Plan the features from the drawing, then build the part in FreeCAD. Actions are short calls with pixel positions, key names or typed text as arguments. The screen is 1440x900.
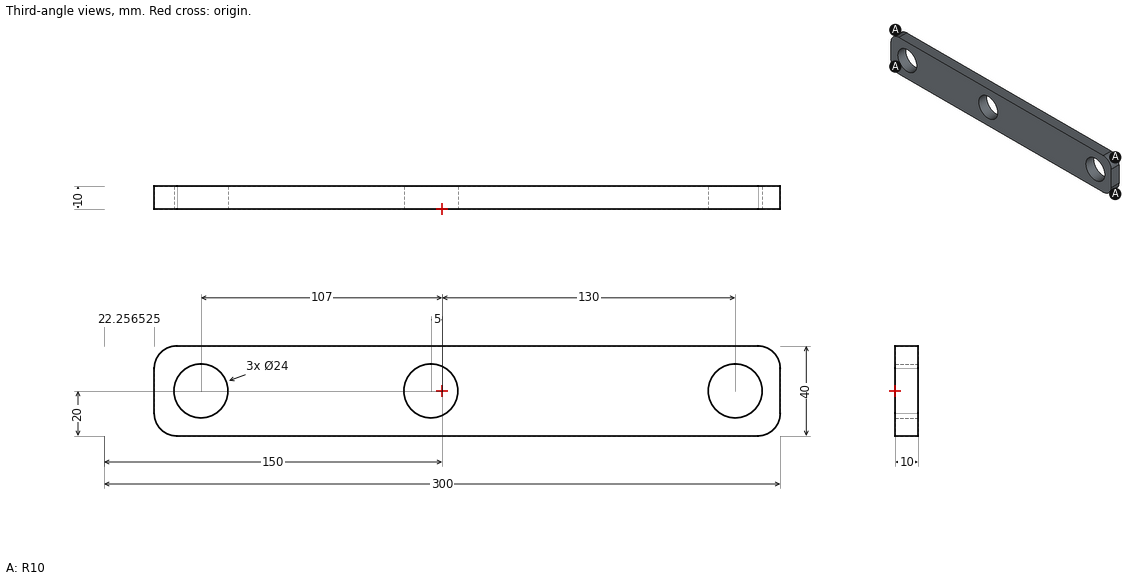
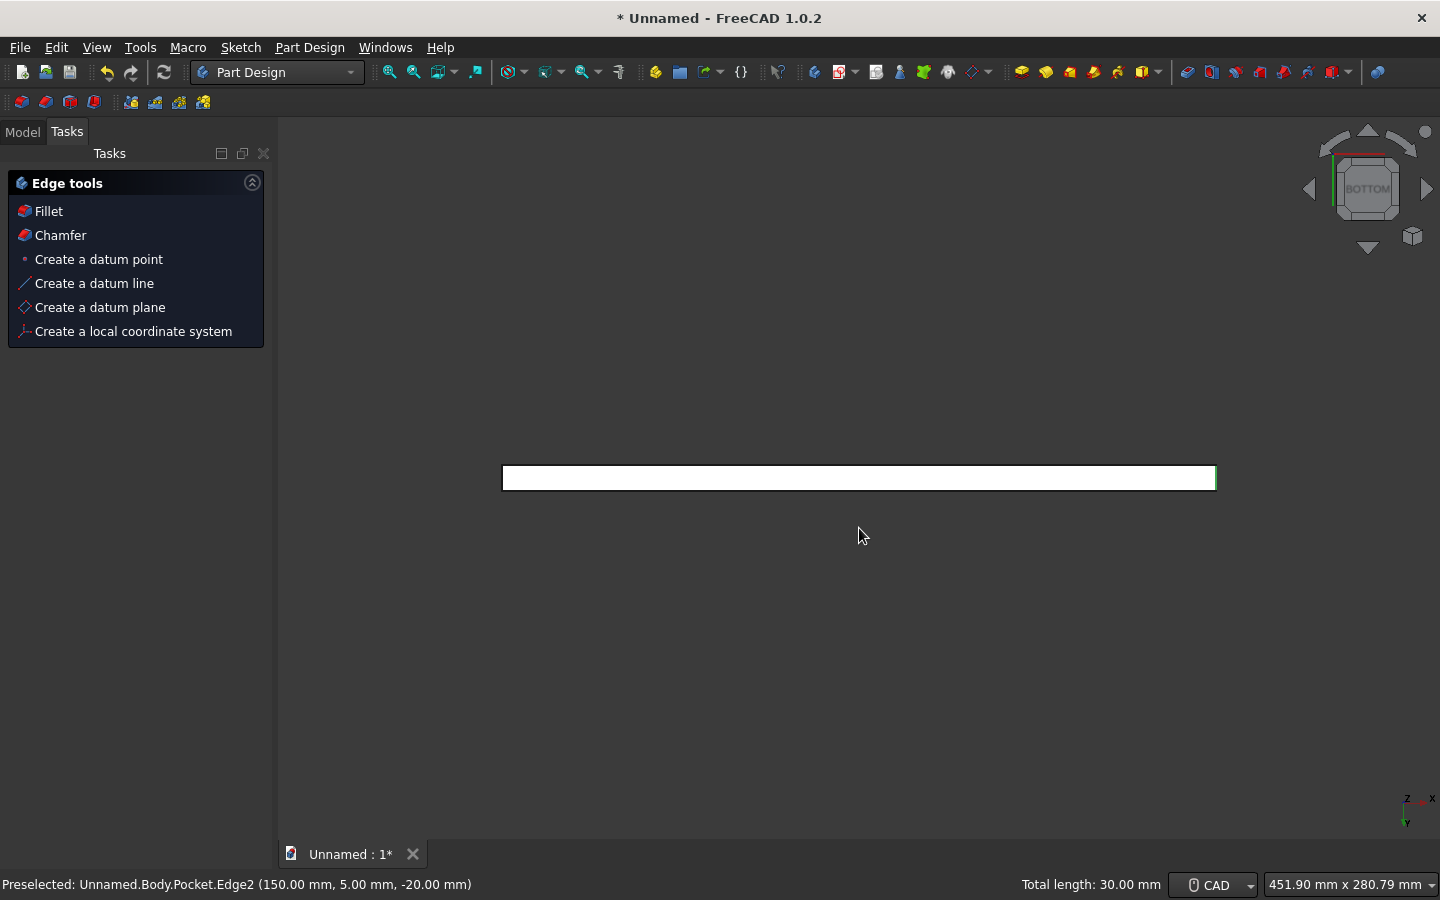
click(502, 477, ctrl)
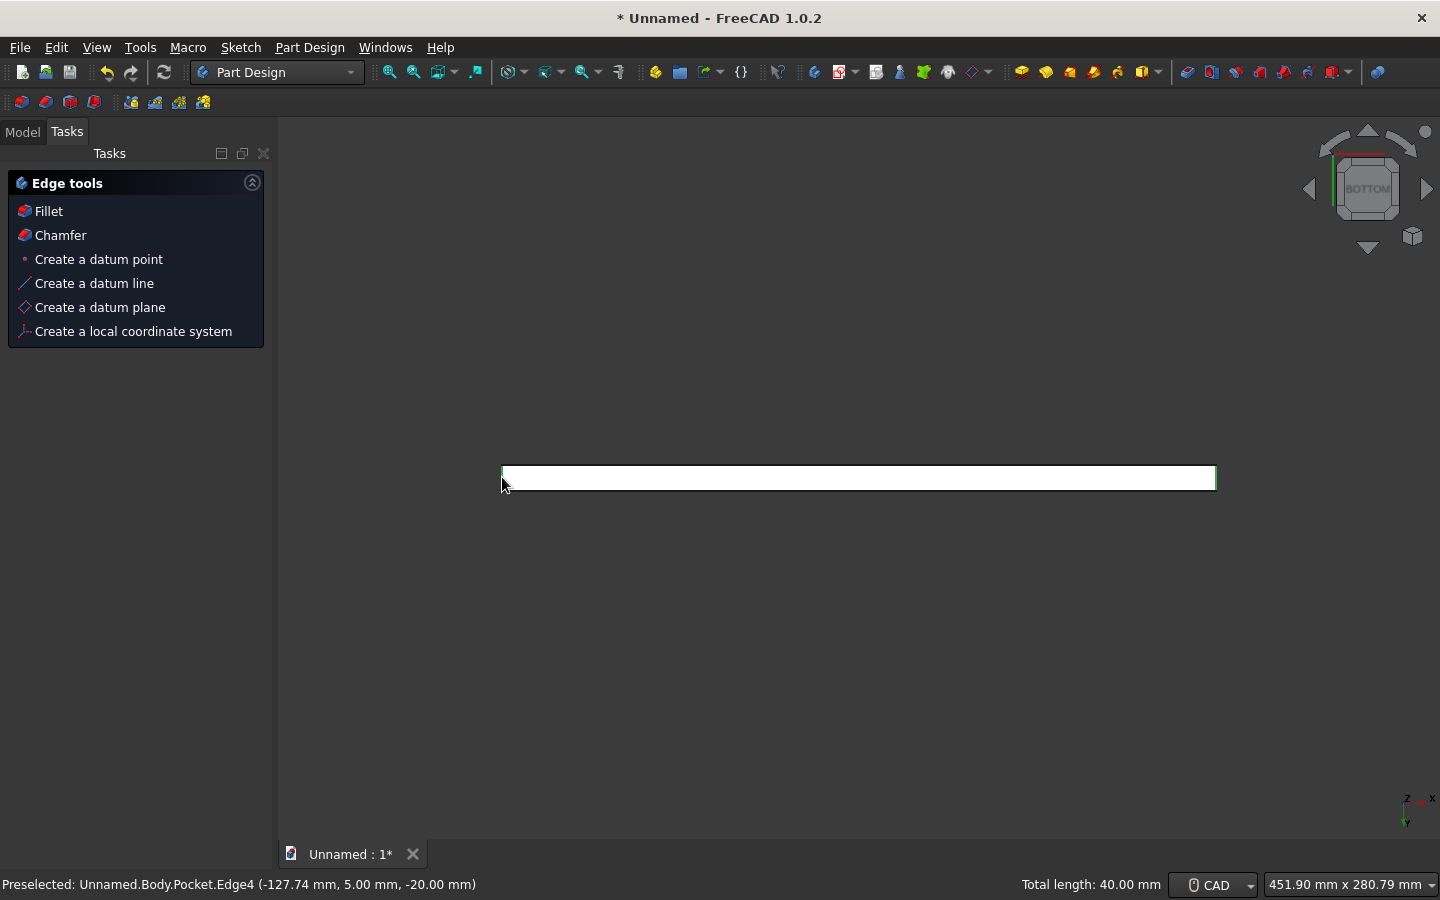
click(22, 102)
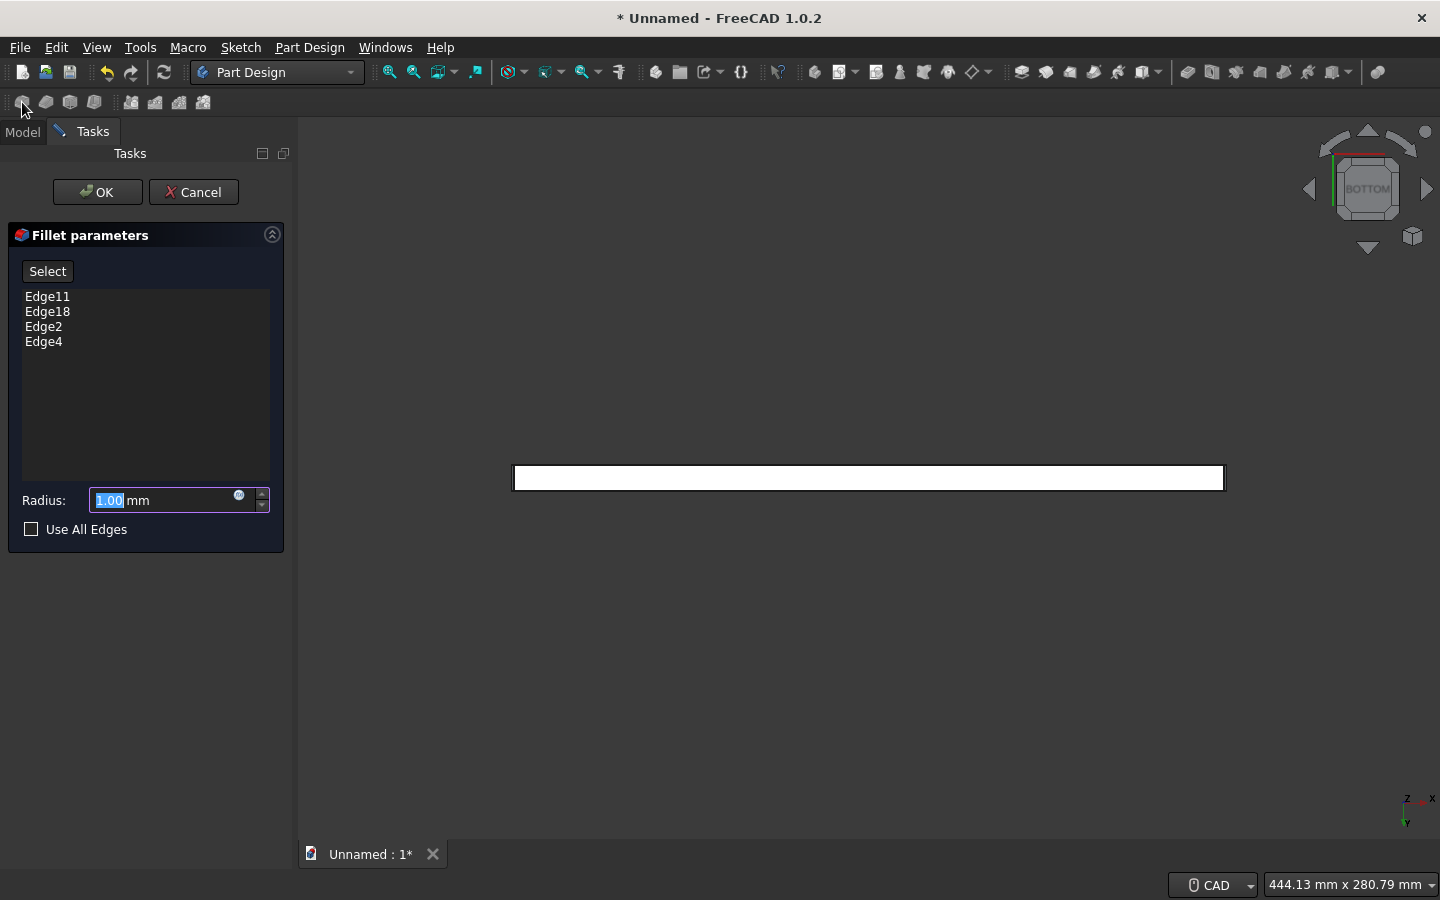
text(10)
key(Tab)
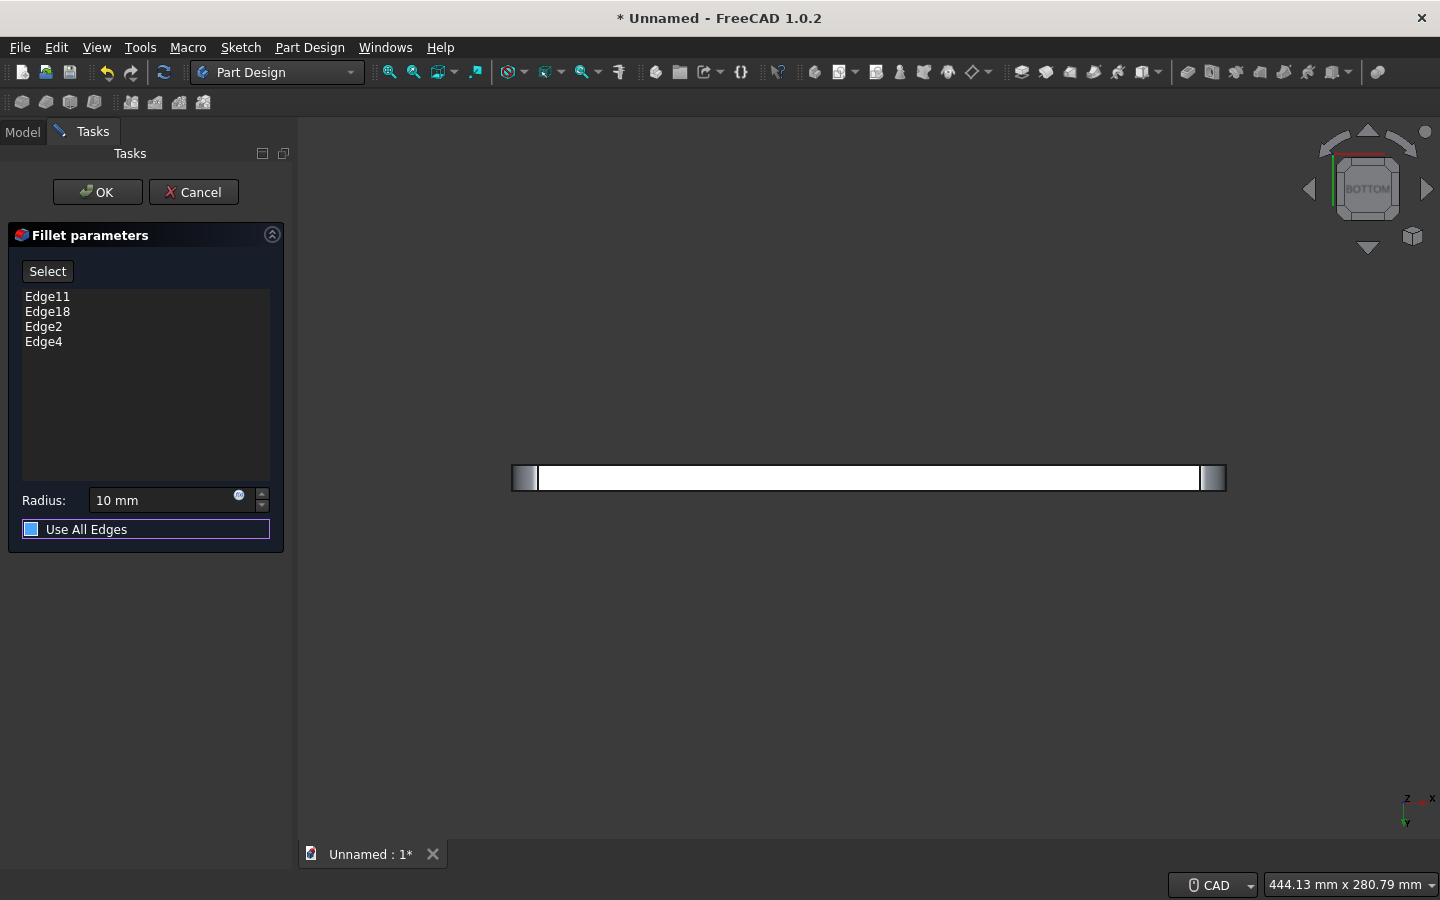
click(98, 192)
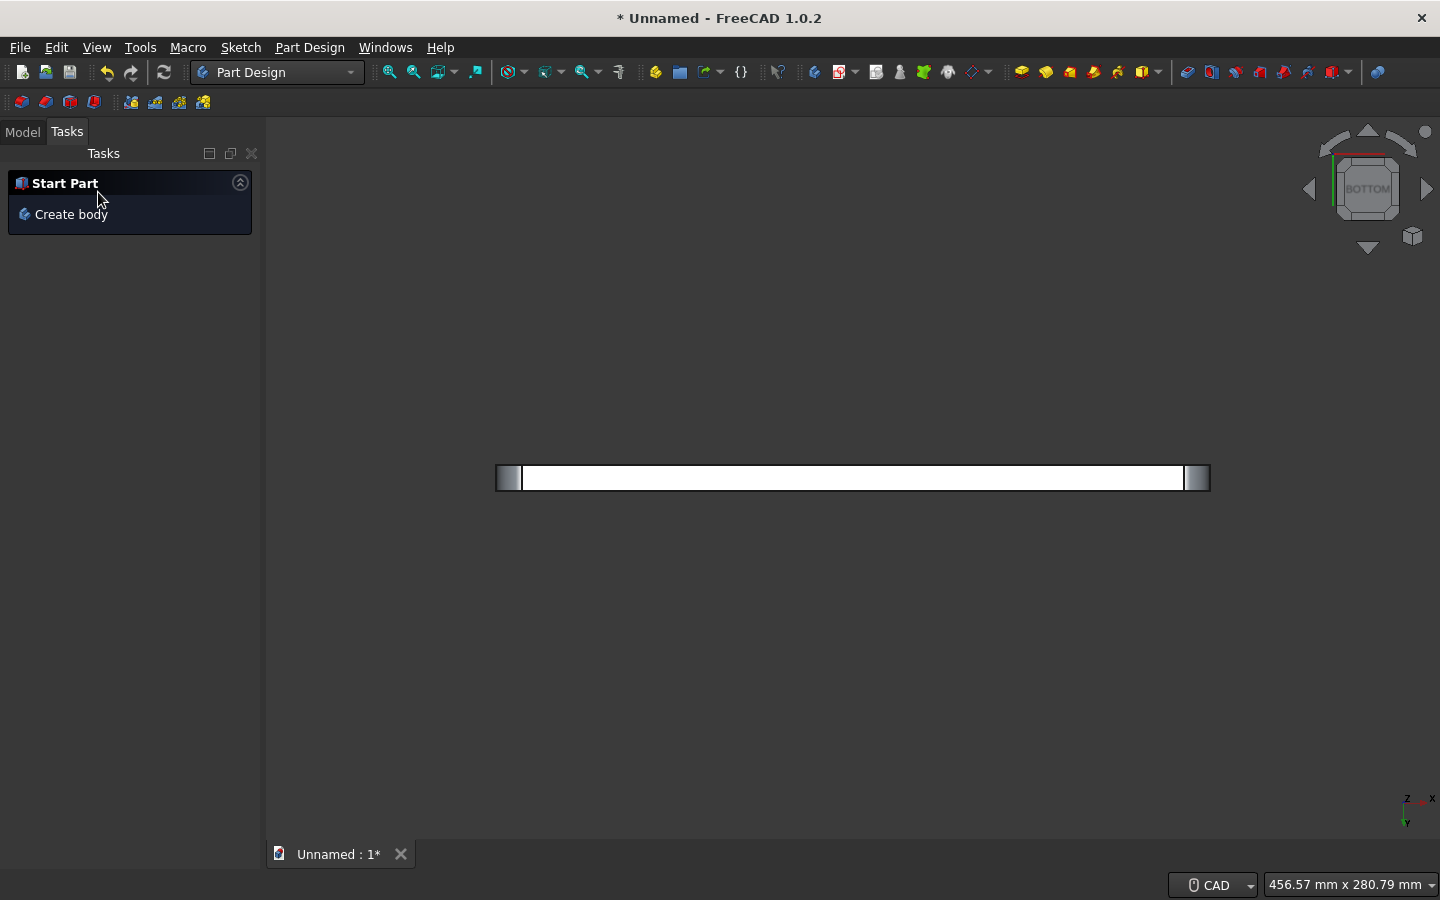
key(0)